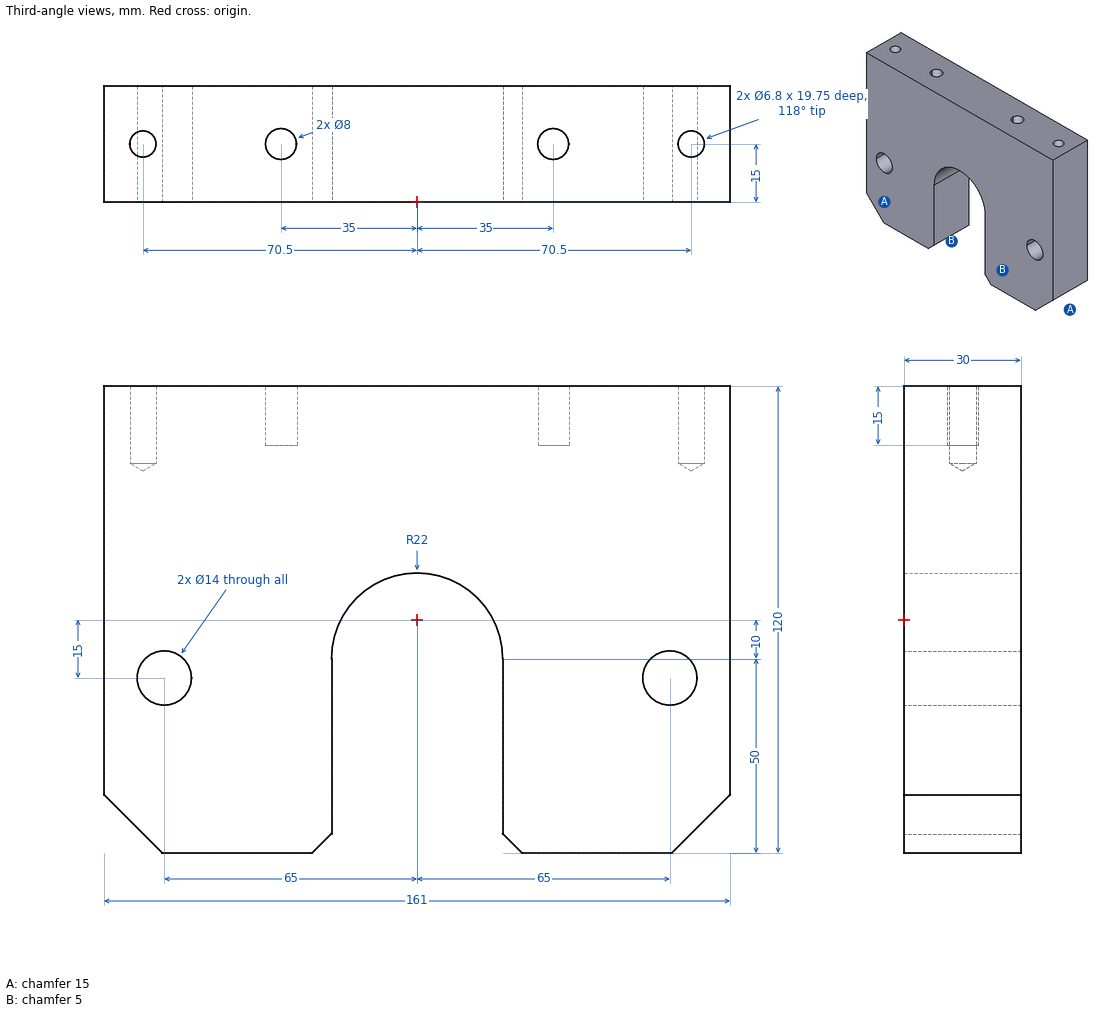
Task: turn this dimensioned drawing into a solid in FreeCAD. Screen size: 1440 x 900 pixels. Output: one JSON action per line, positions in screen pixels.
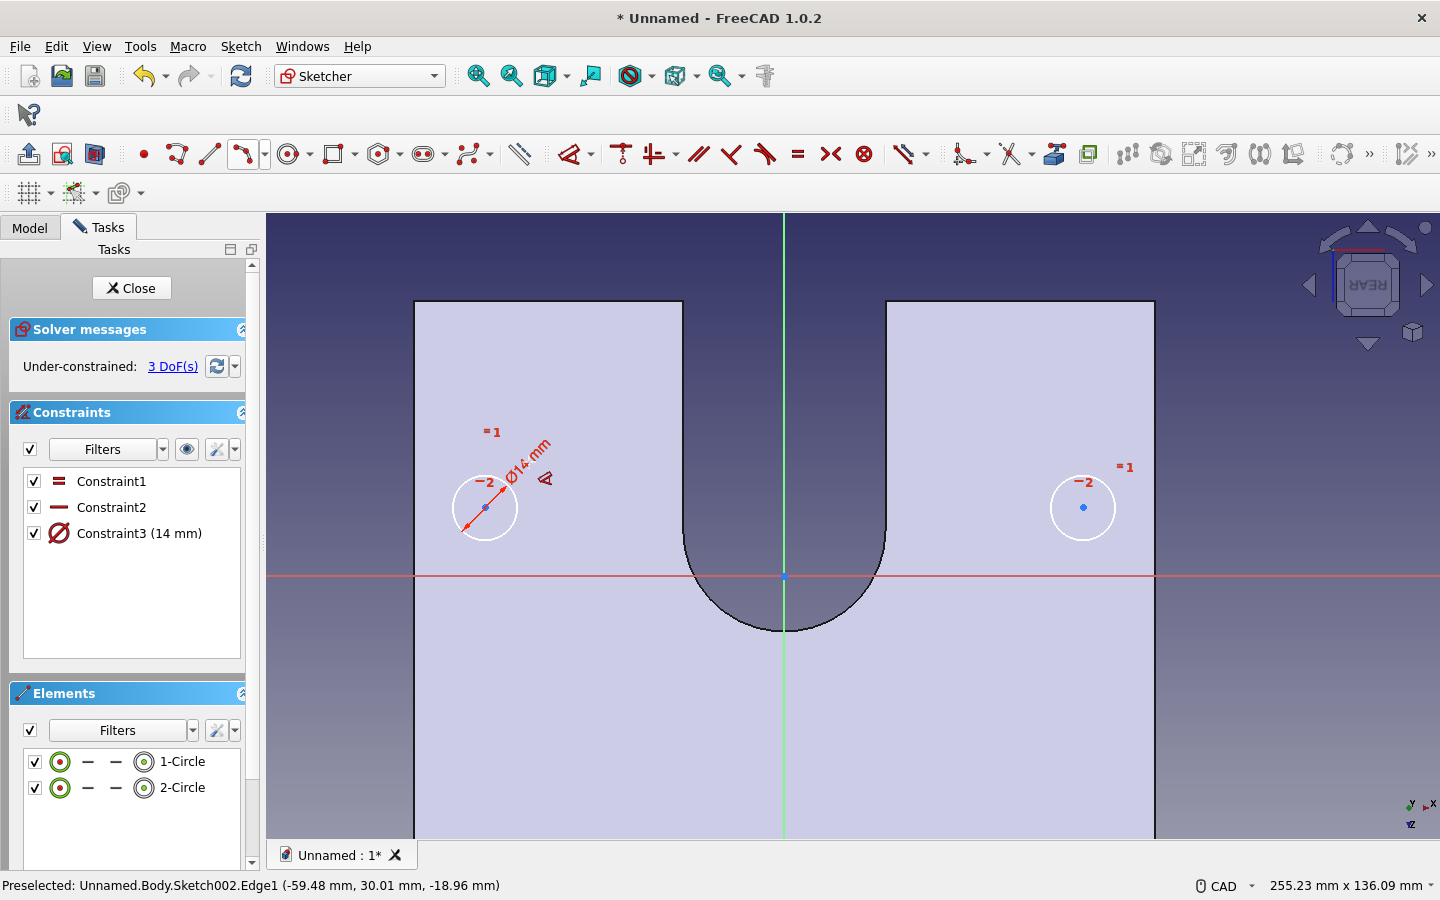
{"action": "left_click", "coordinate": [485, 508]}
{"action": "left_click", "coordinate": [635, 610]}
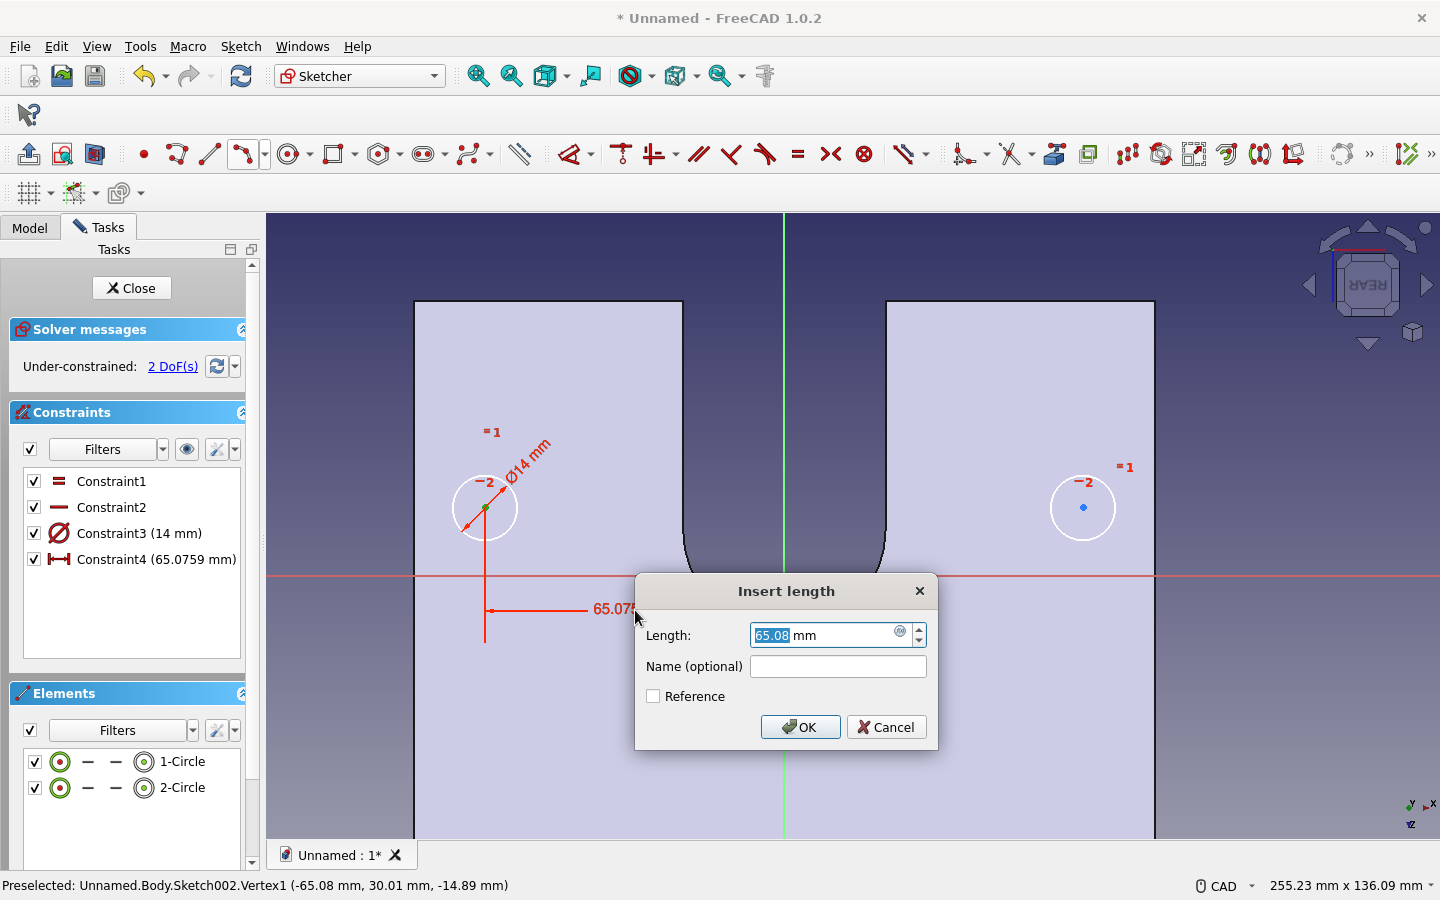
{"action": "type", "text": "65"}
{"action": "key", "text": "Return"}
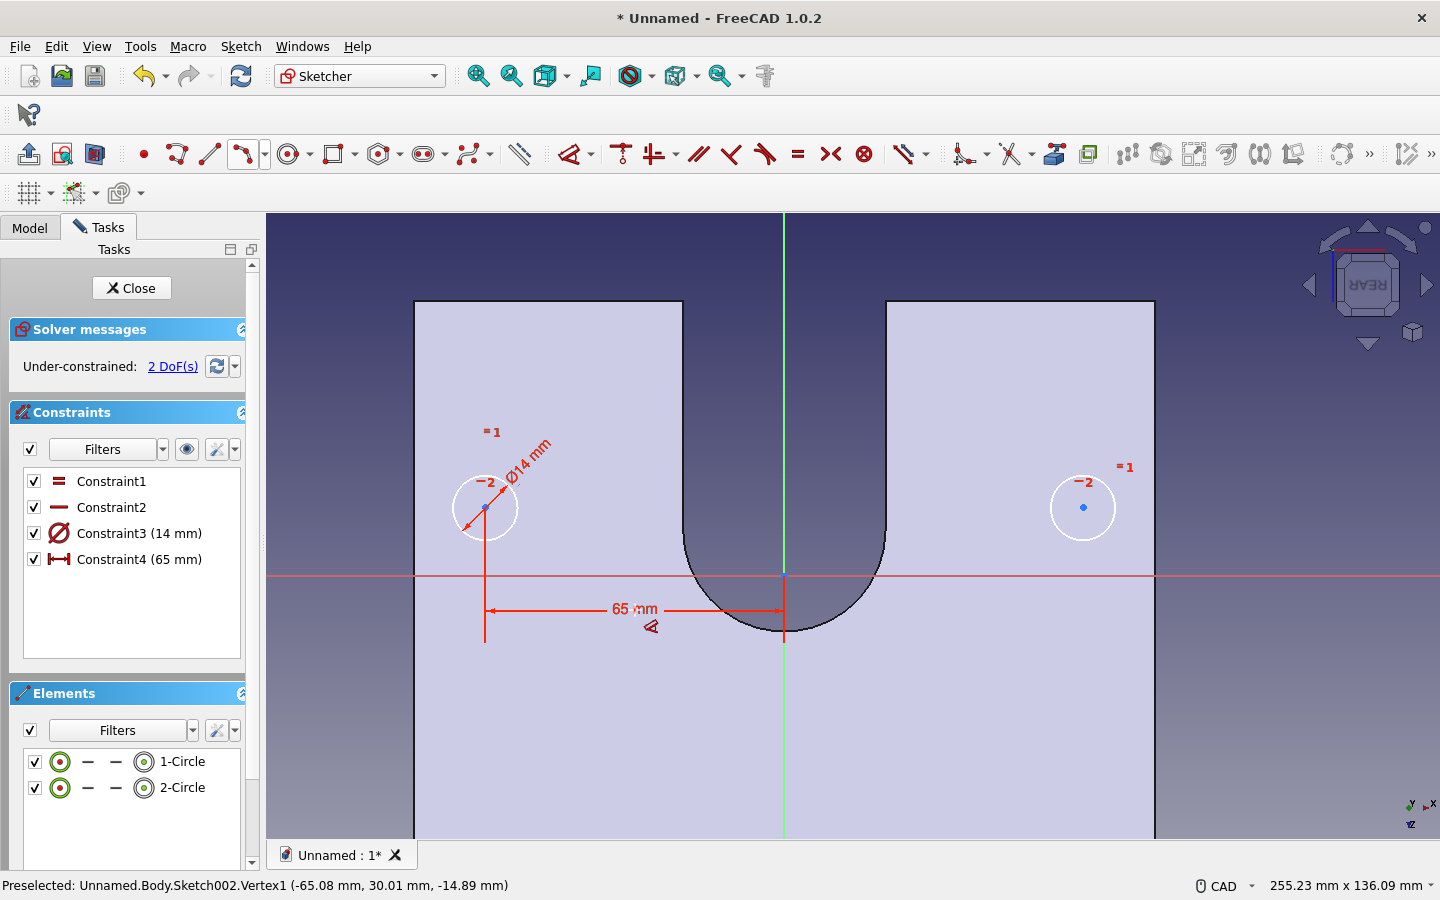
{"action": "left_click", "coordinate": [485, 508]}
{"action": "left_click", "coordinate": [451, 542]}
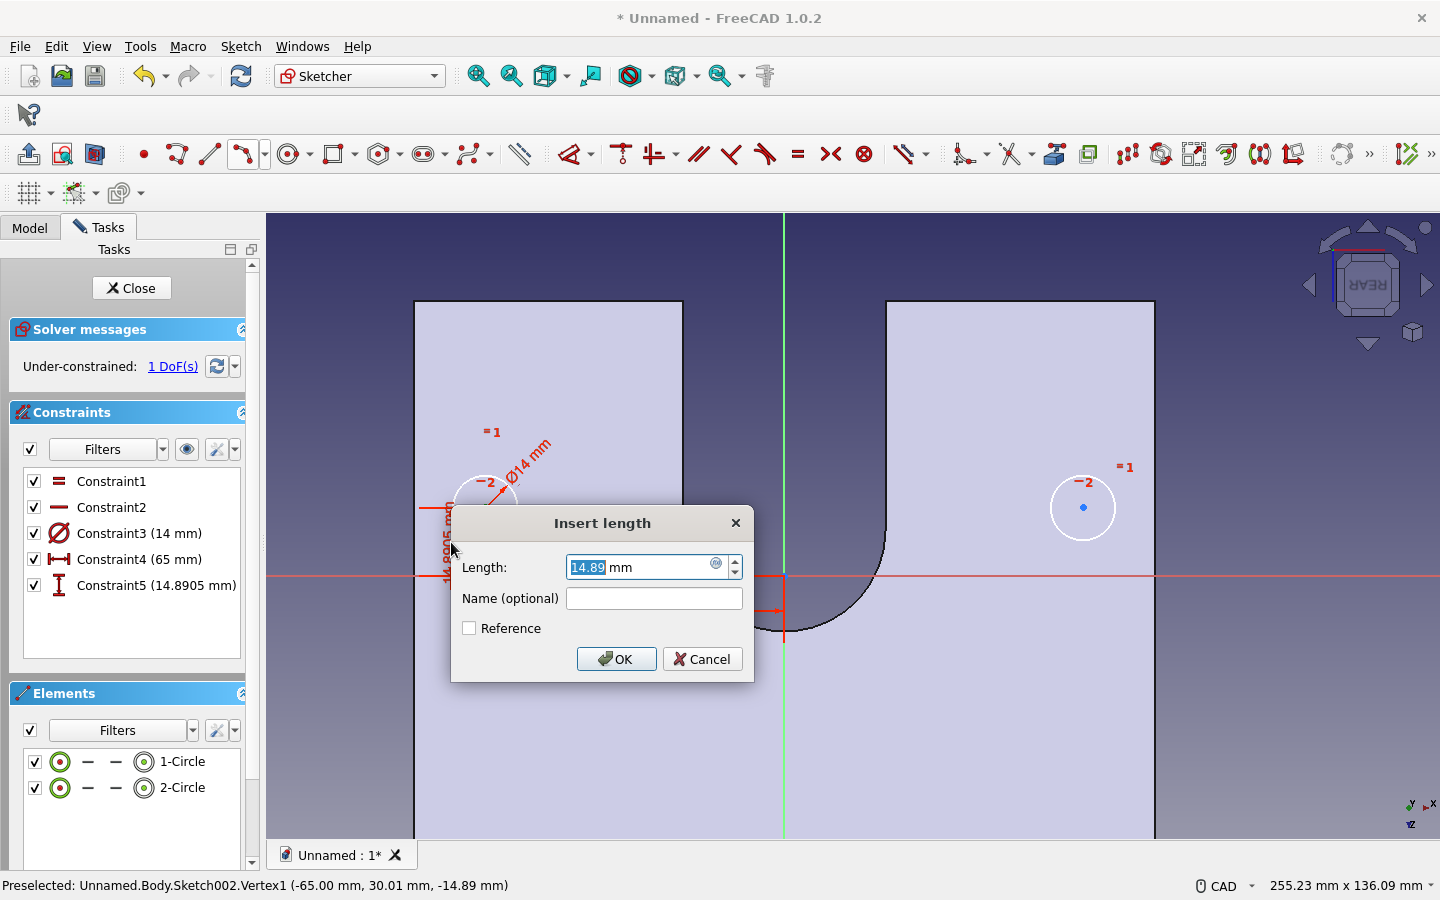
{"action": "type", "text": "15"}
{"action": "key", "text": "Return"}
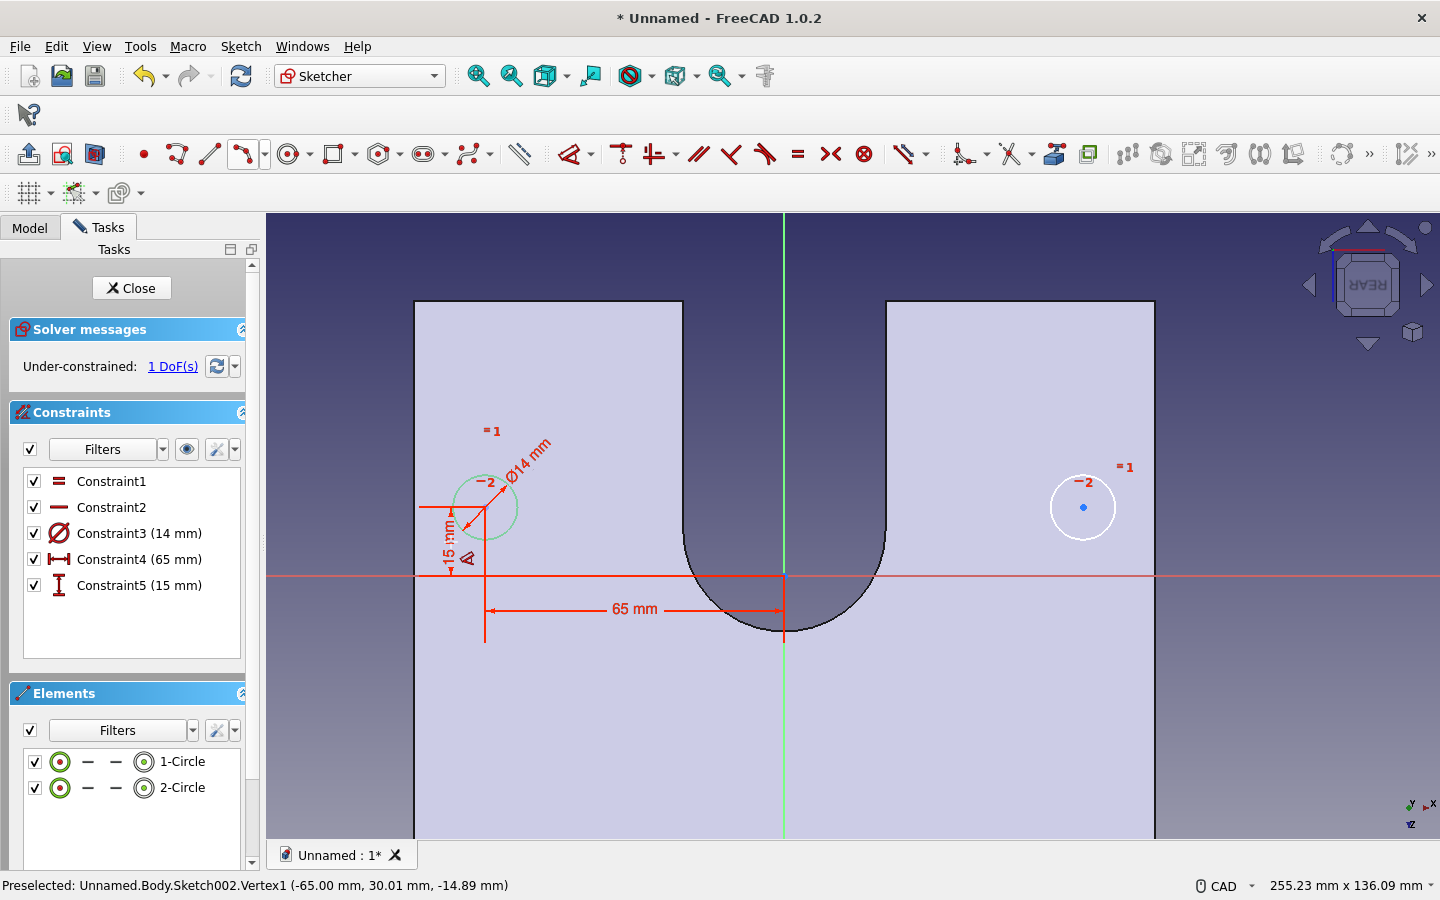
{"action": "left_click", "coordinate": [1083, 507]}
{"action": "left_click", "coordinate": [934, 610]}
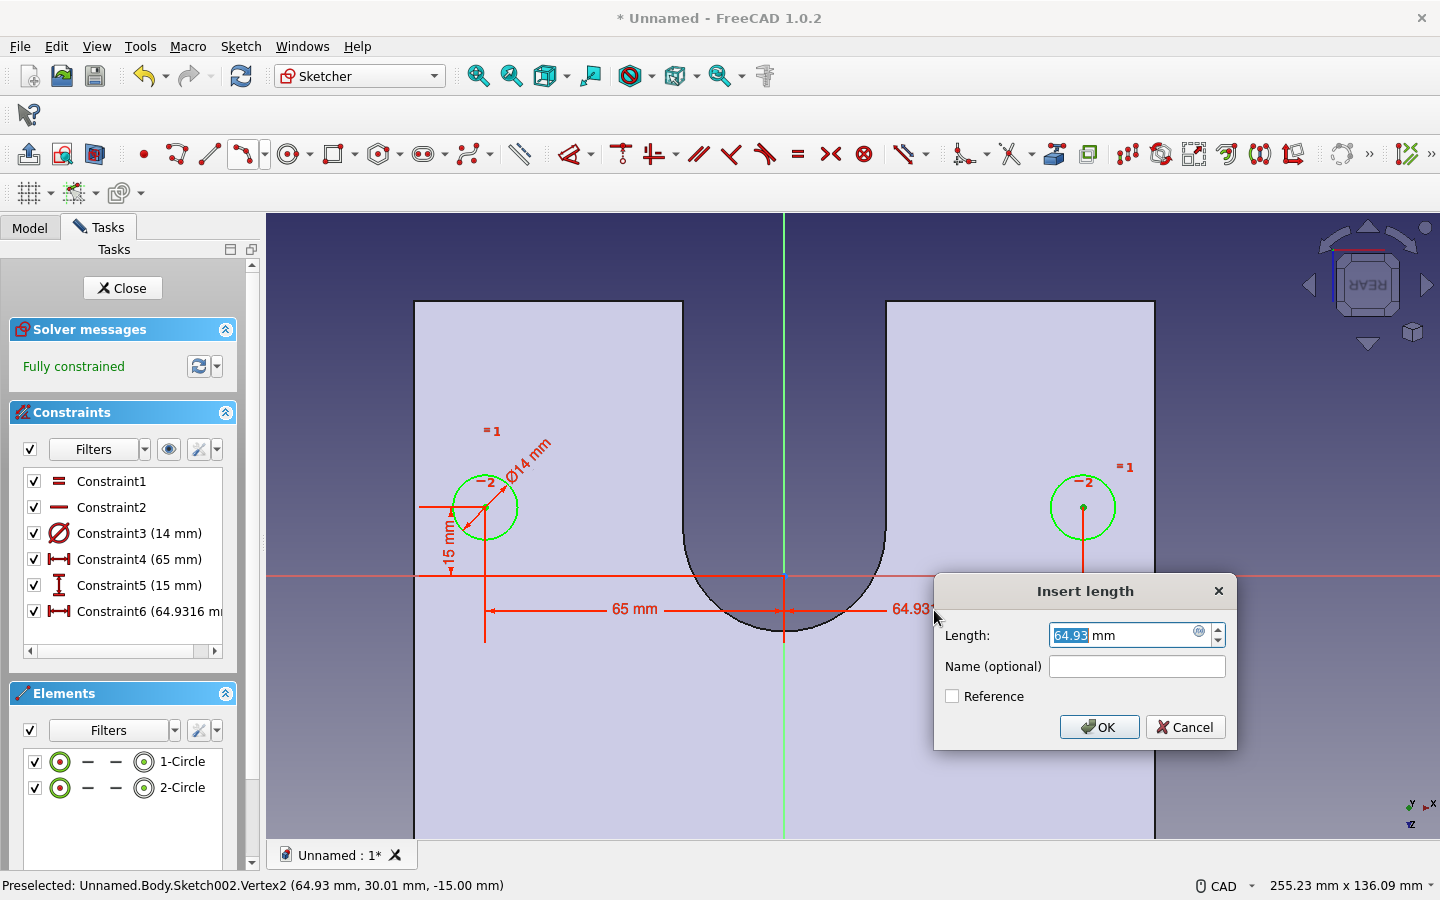
{"action": "type", "text": "65"}
{"action": "key", "text": "Return"}
{"action": "key", "text": "Escape"}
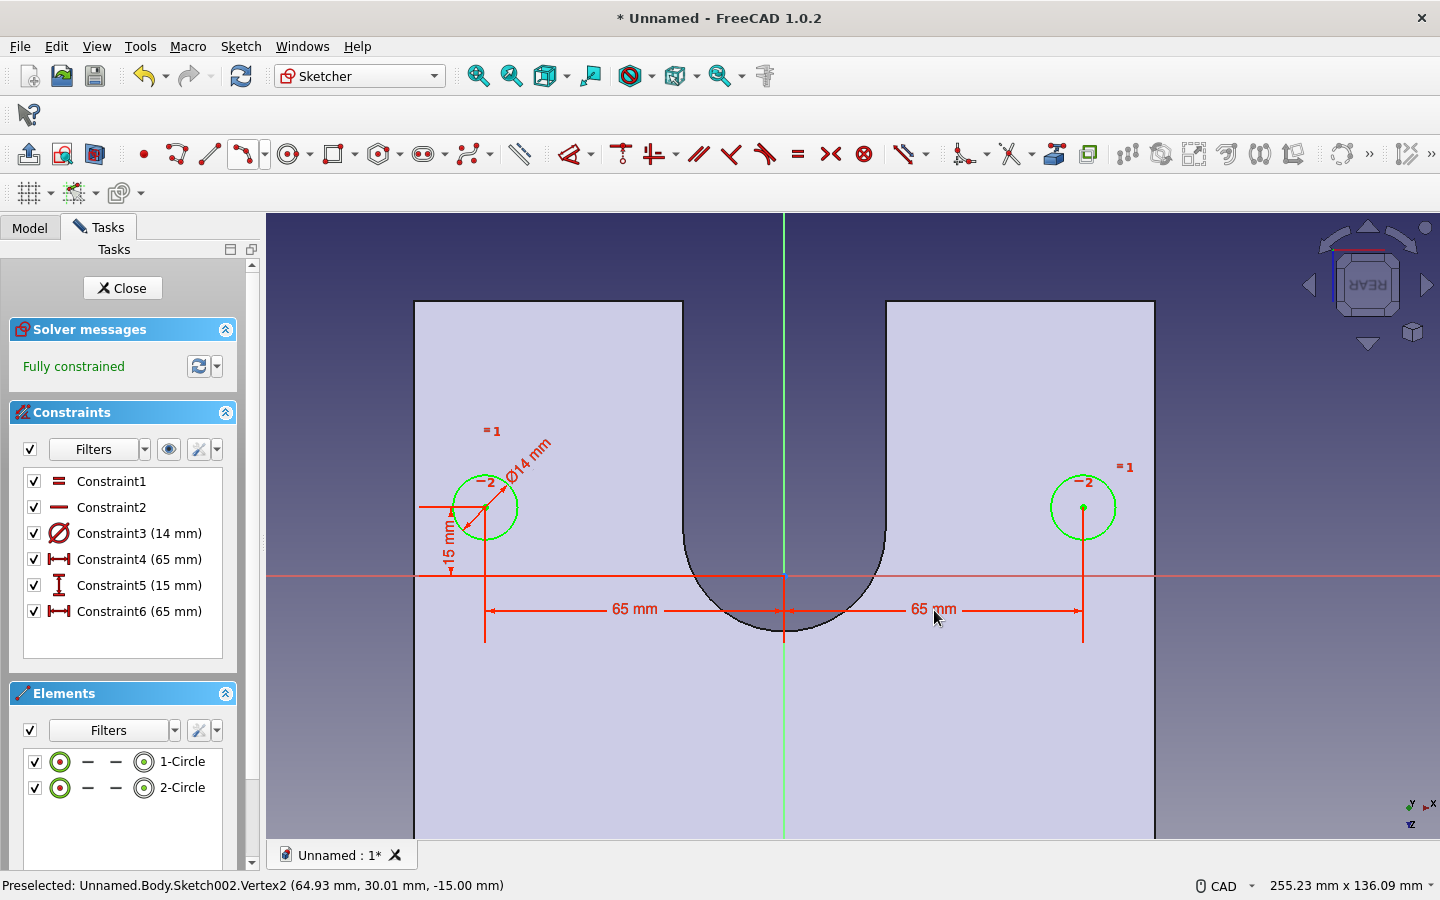
{"action": "left_click", "coordinate": [123, 288]}